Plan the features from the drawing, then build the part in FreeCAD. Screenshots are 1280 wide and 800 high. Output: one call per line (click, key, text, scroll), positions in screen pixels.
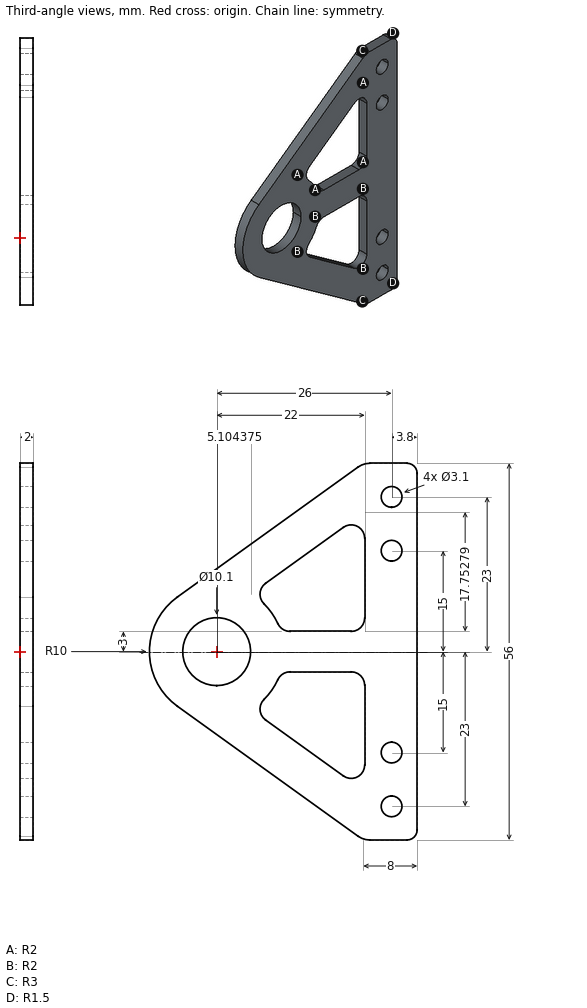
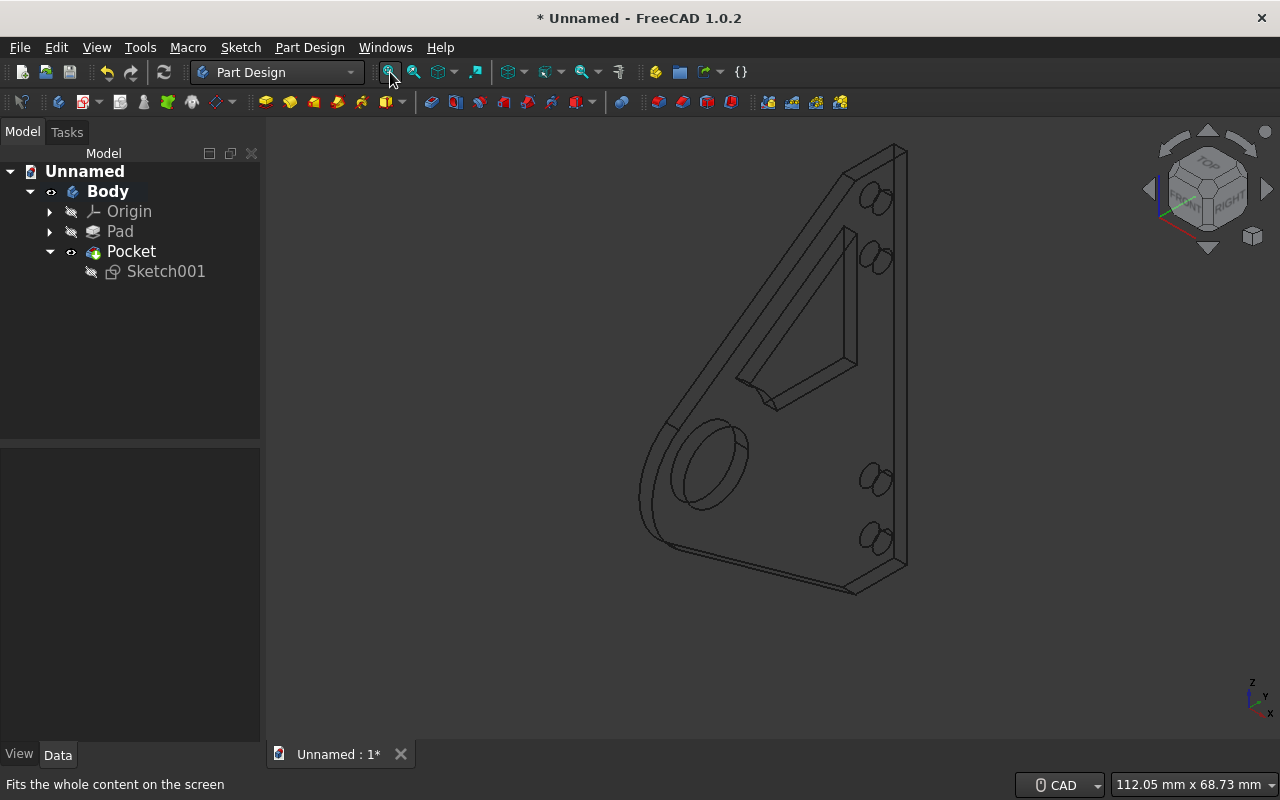
click(850, 360)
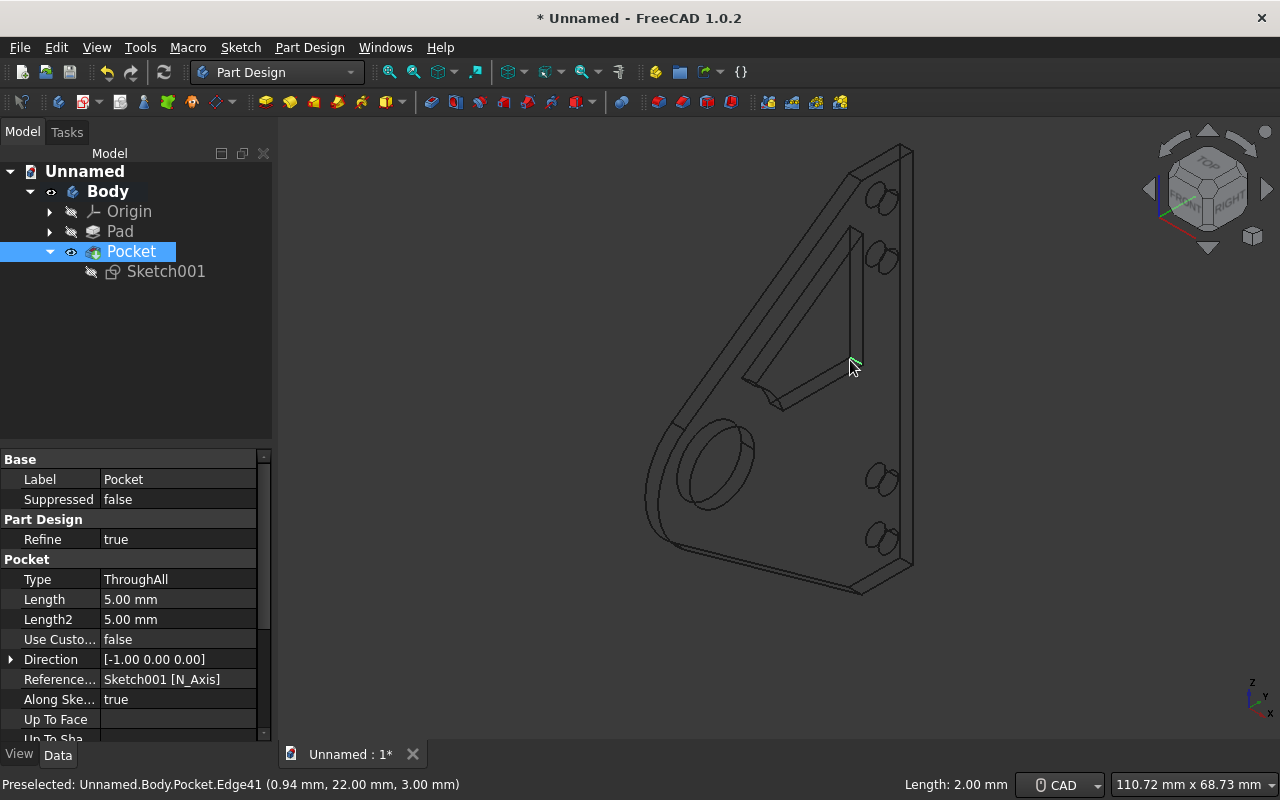
click(856, 229, ctrl)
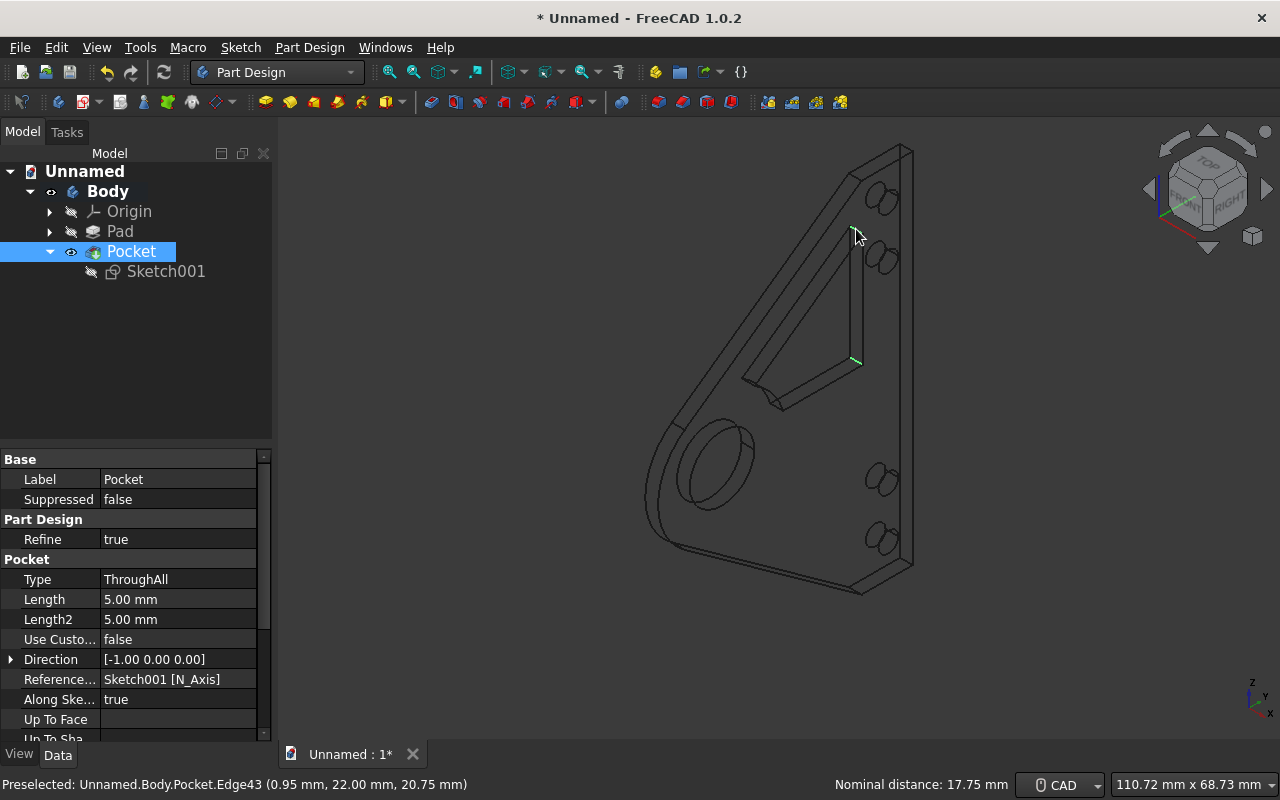
click(748, 381, ctrl)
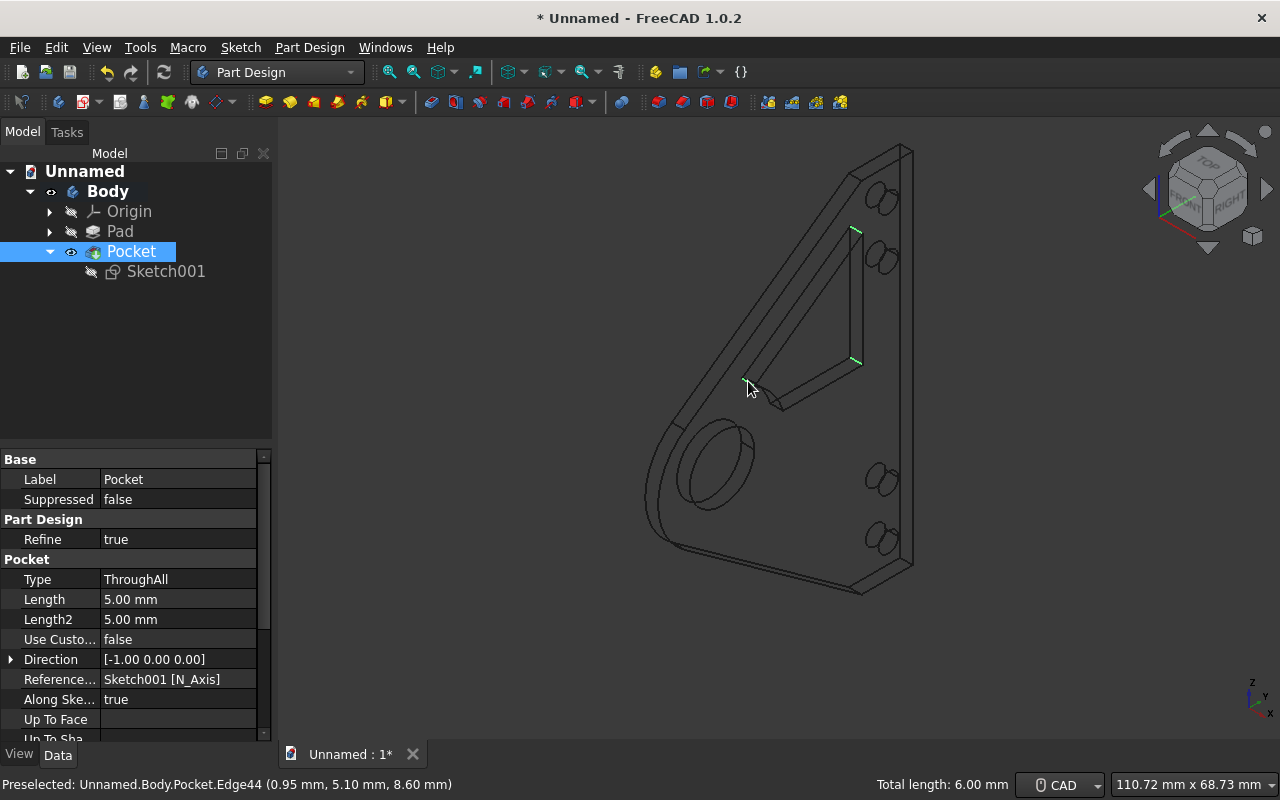
click(774, 405, ctrl)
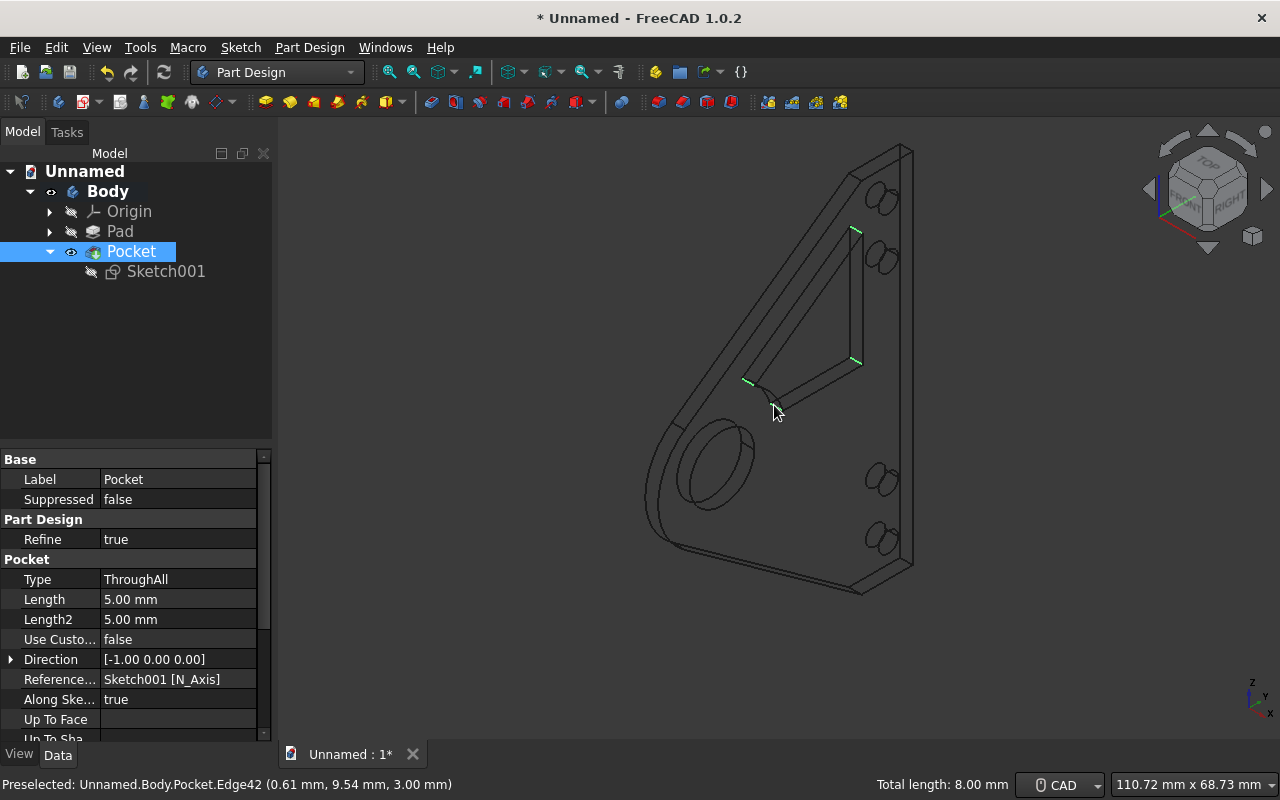
key(v)
key(1)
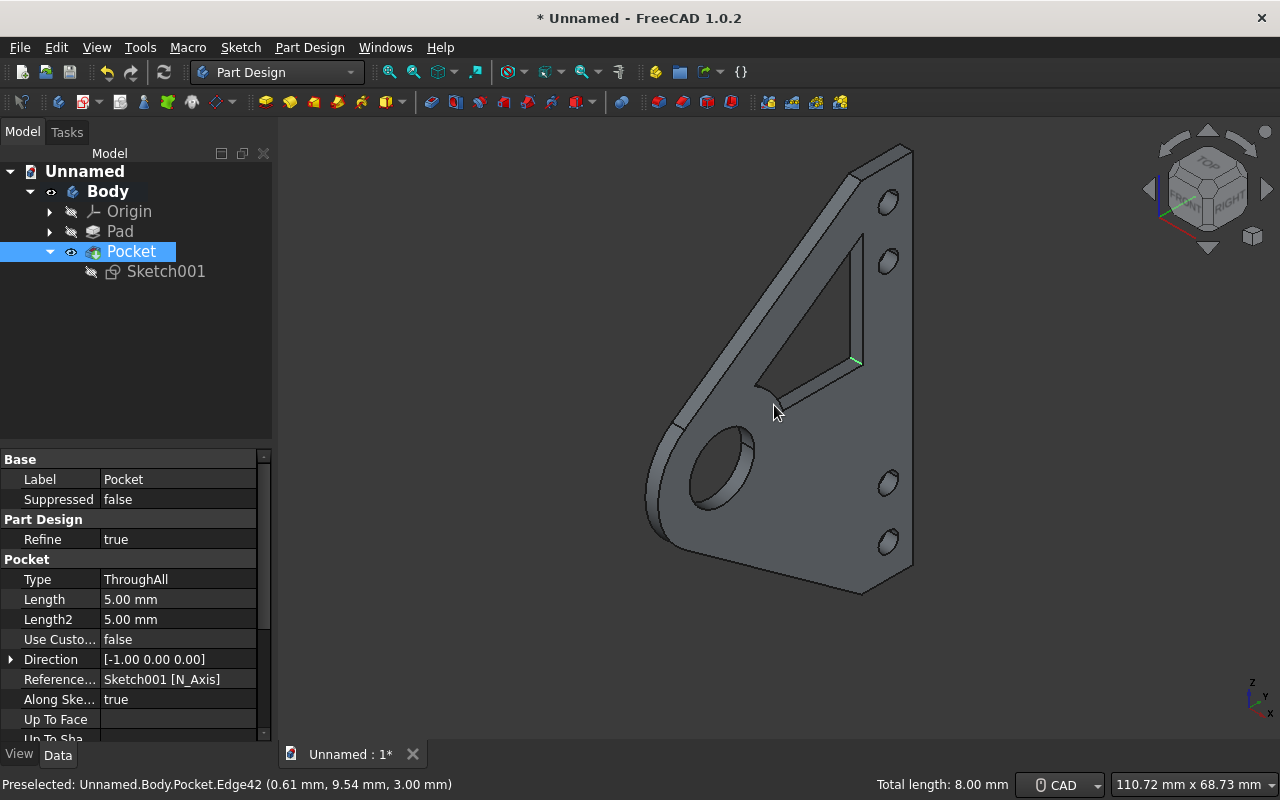
click(660, 102)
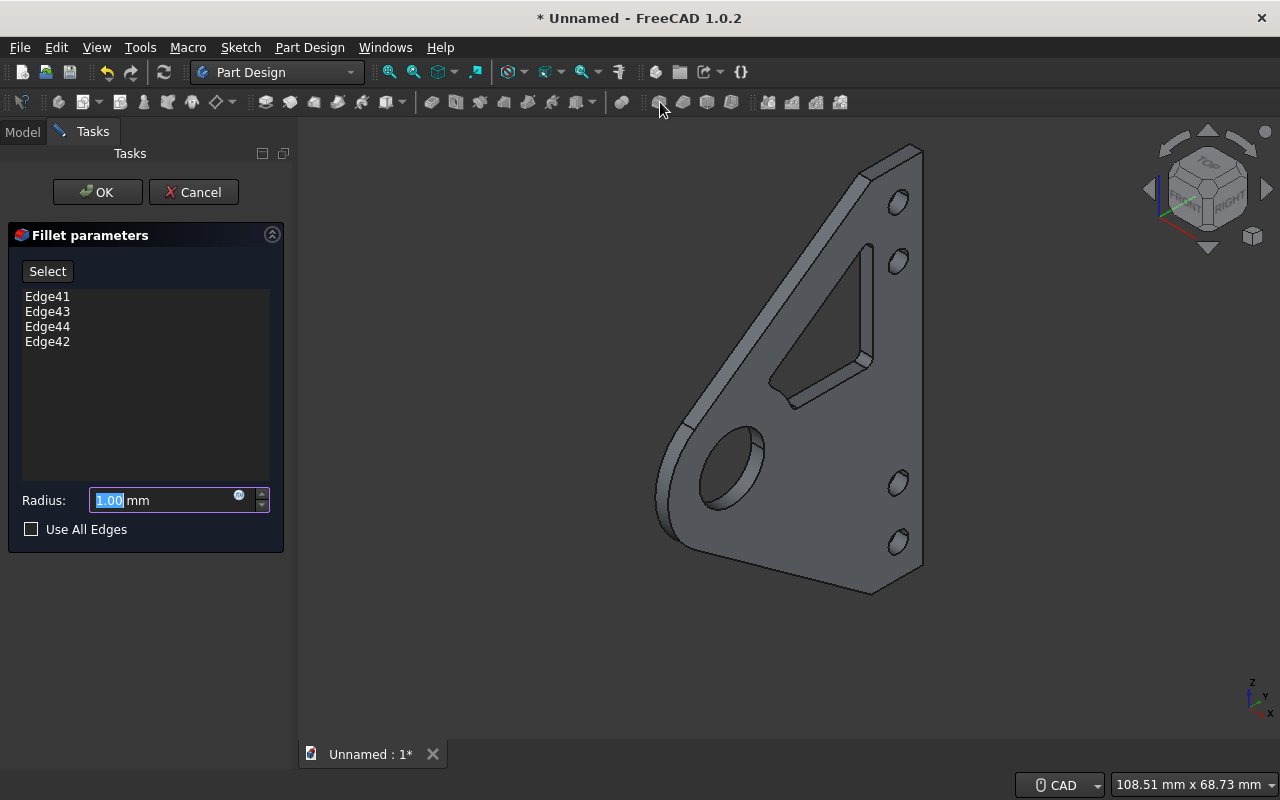
text(2)
key(Tab)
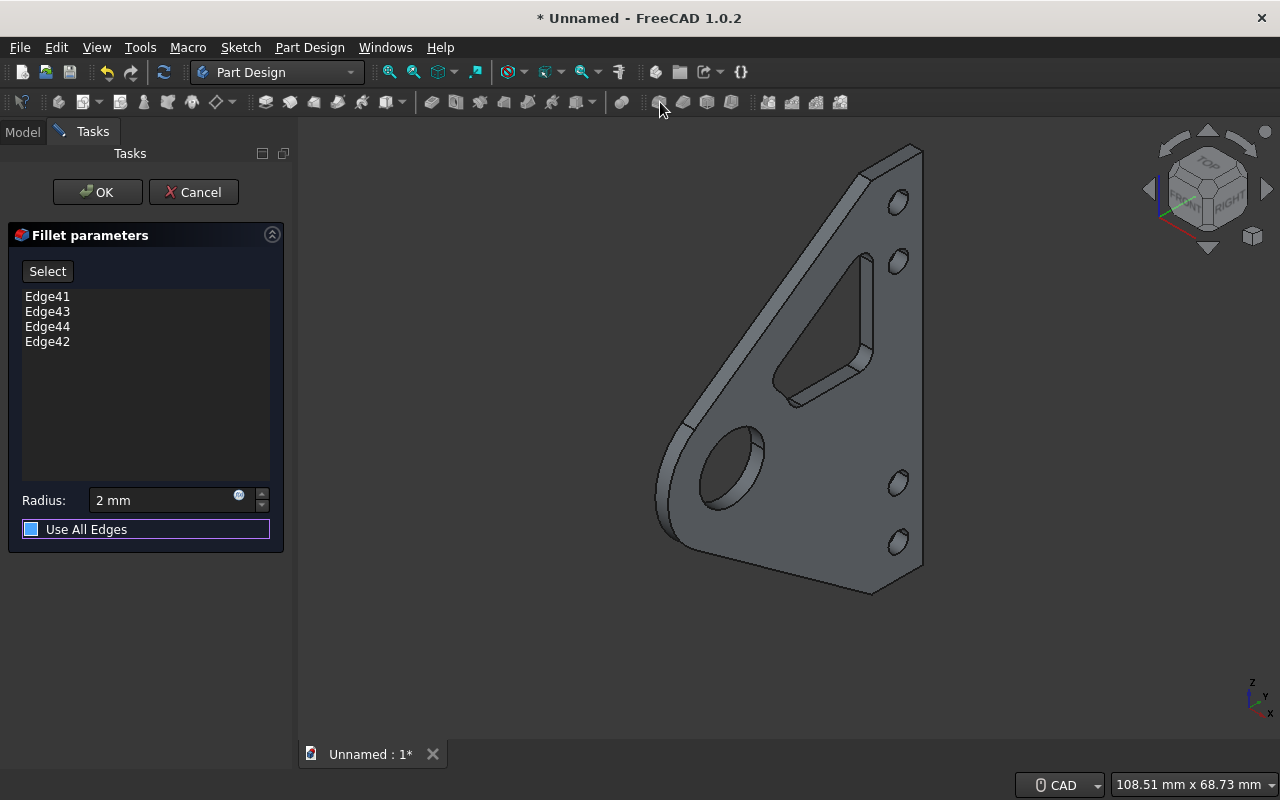
click(98, 192)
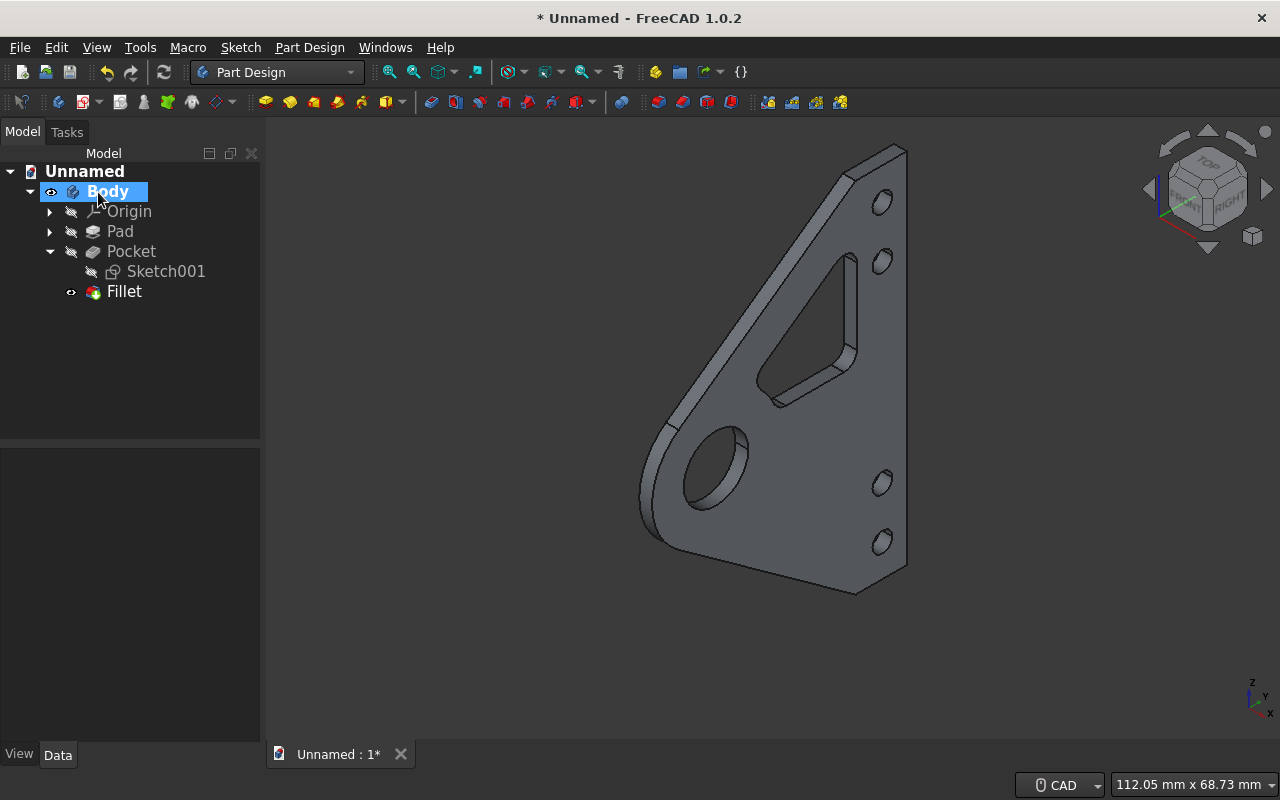
click(116, 252)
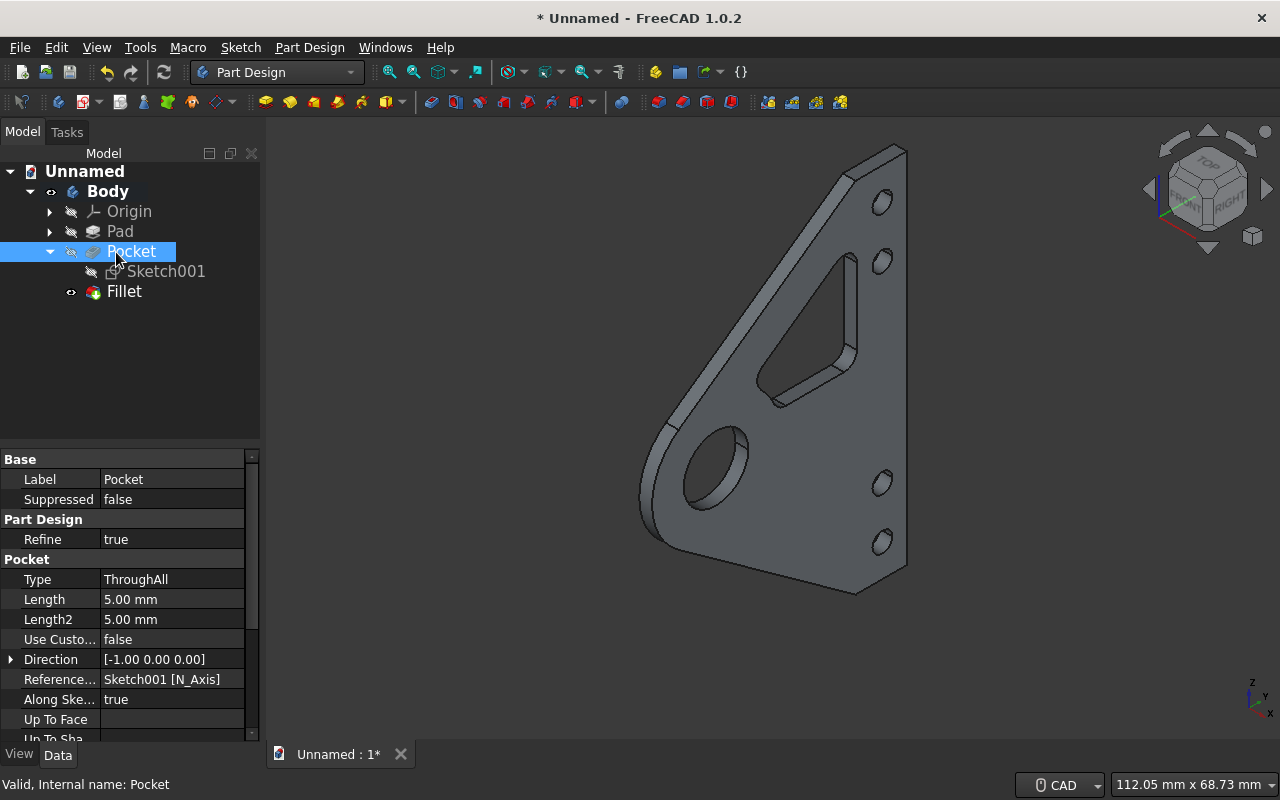
click(768, 102)